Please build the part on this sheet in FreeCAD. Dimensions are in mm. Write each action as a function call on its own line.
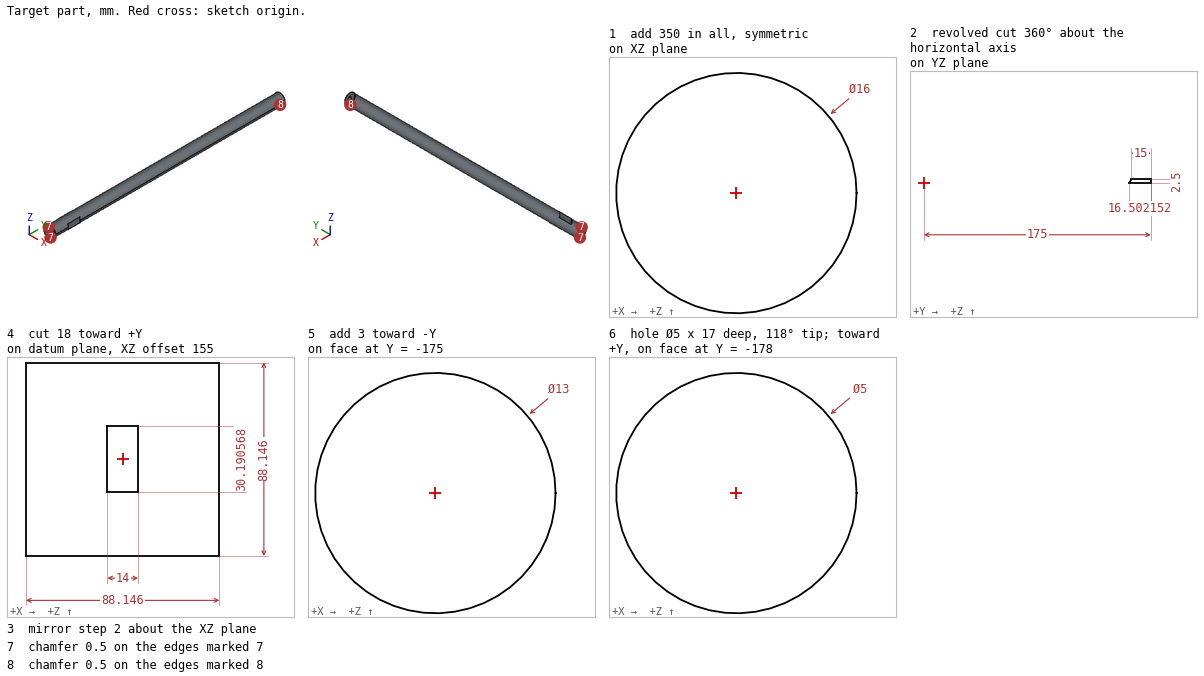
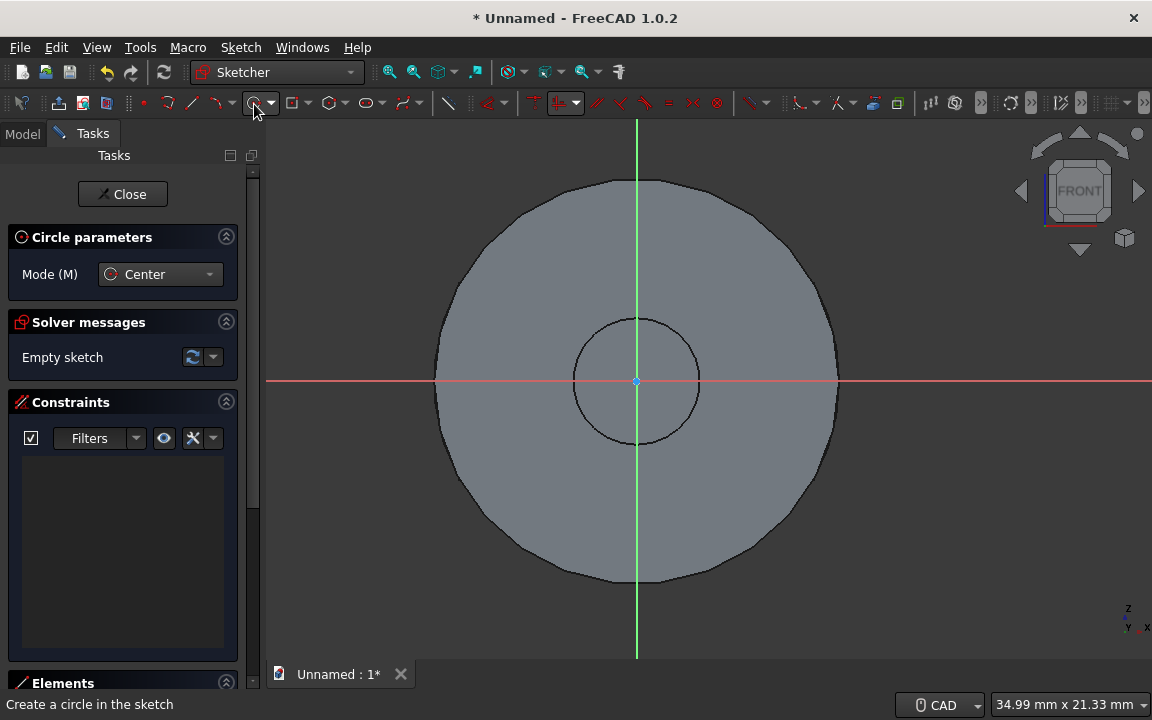
click(637, 381)
move(753, 265)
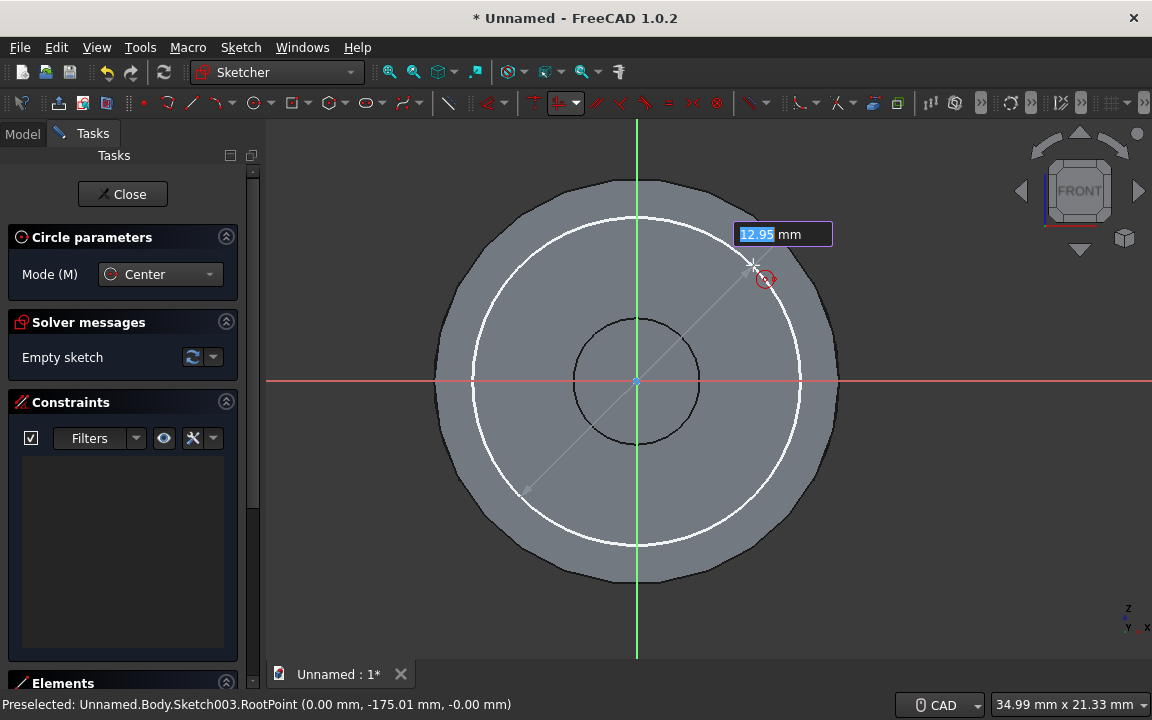
text(13)
key(Return)
key(Escape)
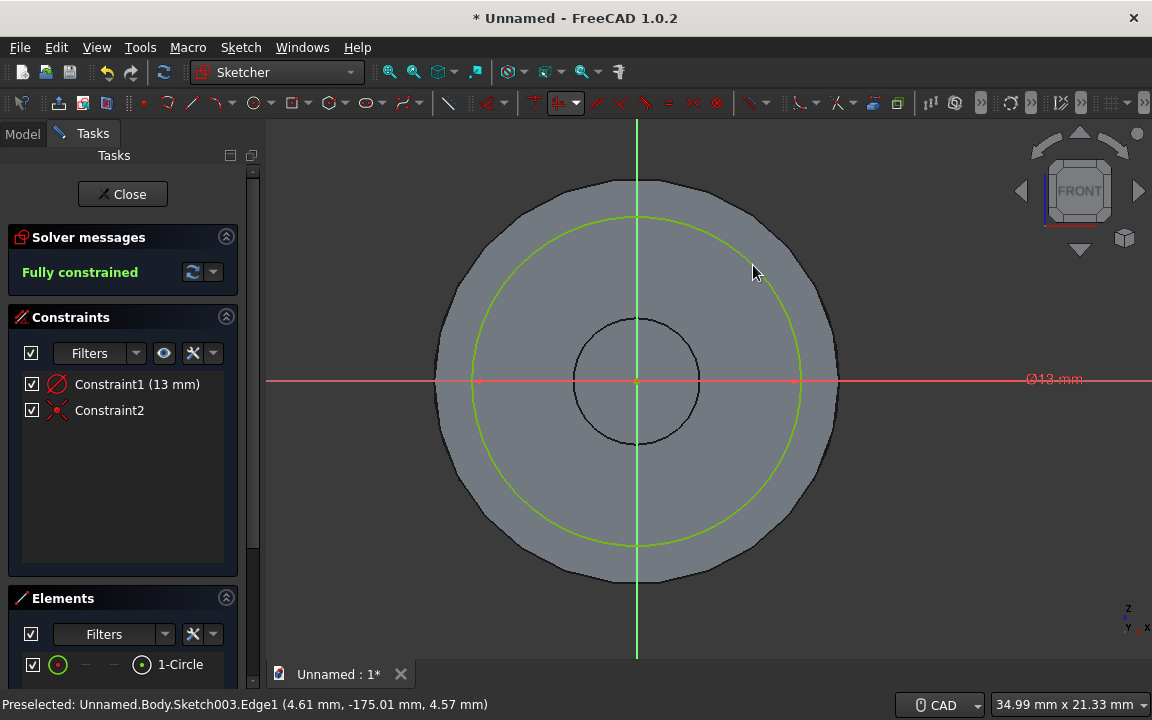
click(123, 194)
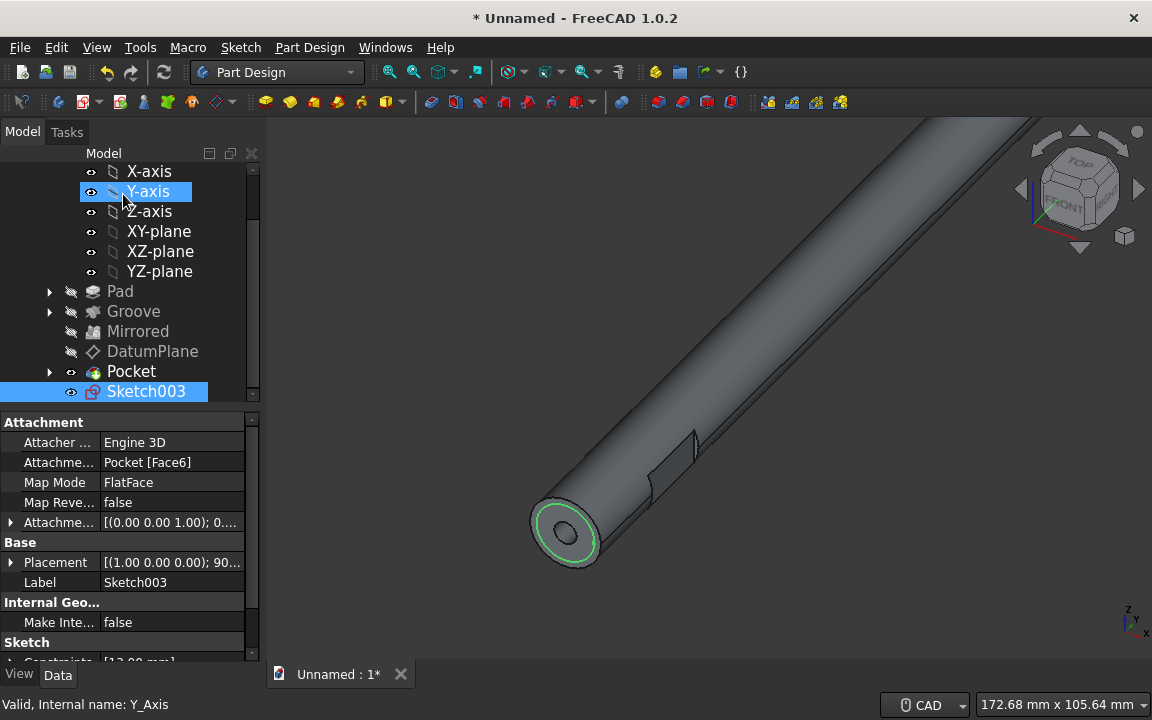
click(266, 102)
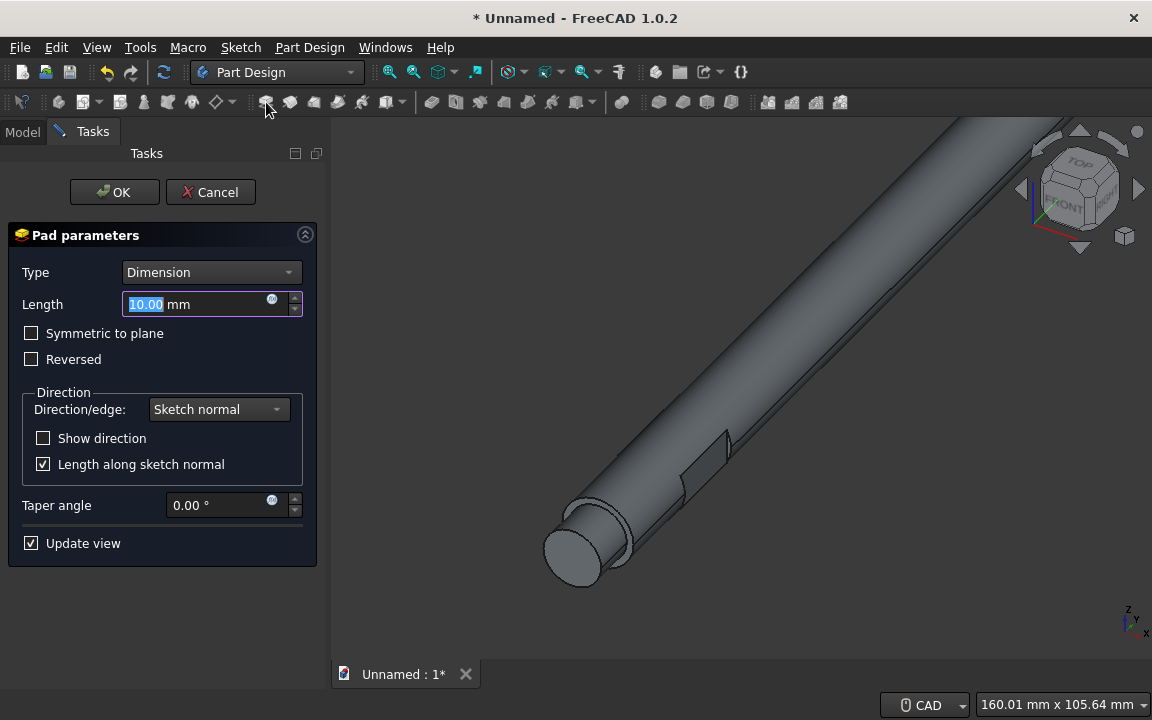
text(3)
key(Tab)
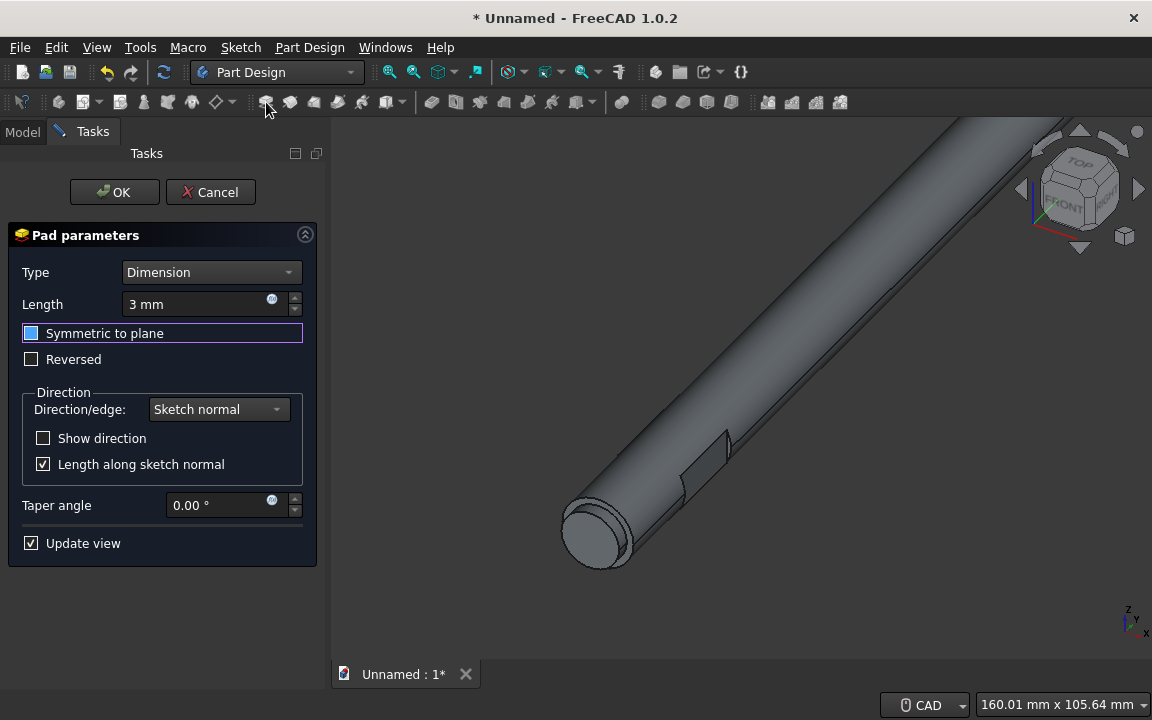
click(115, 192)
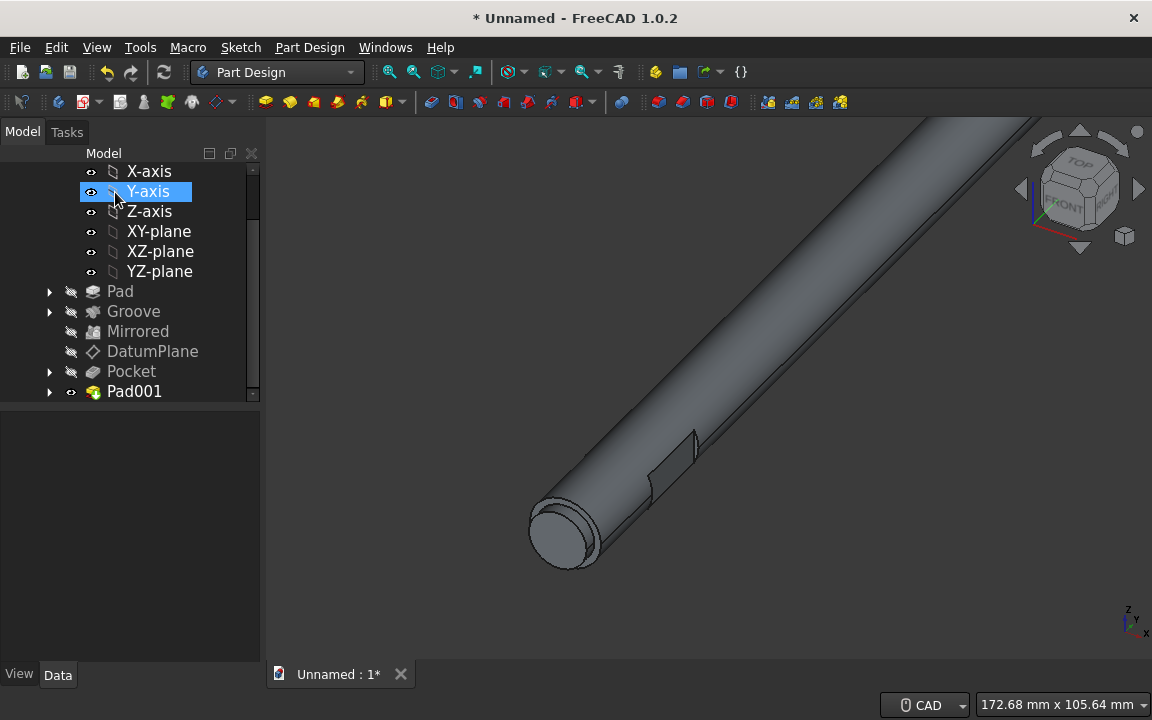
click(390, 72)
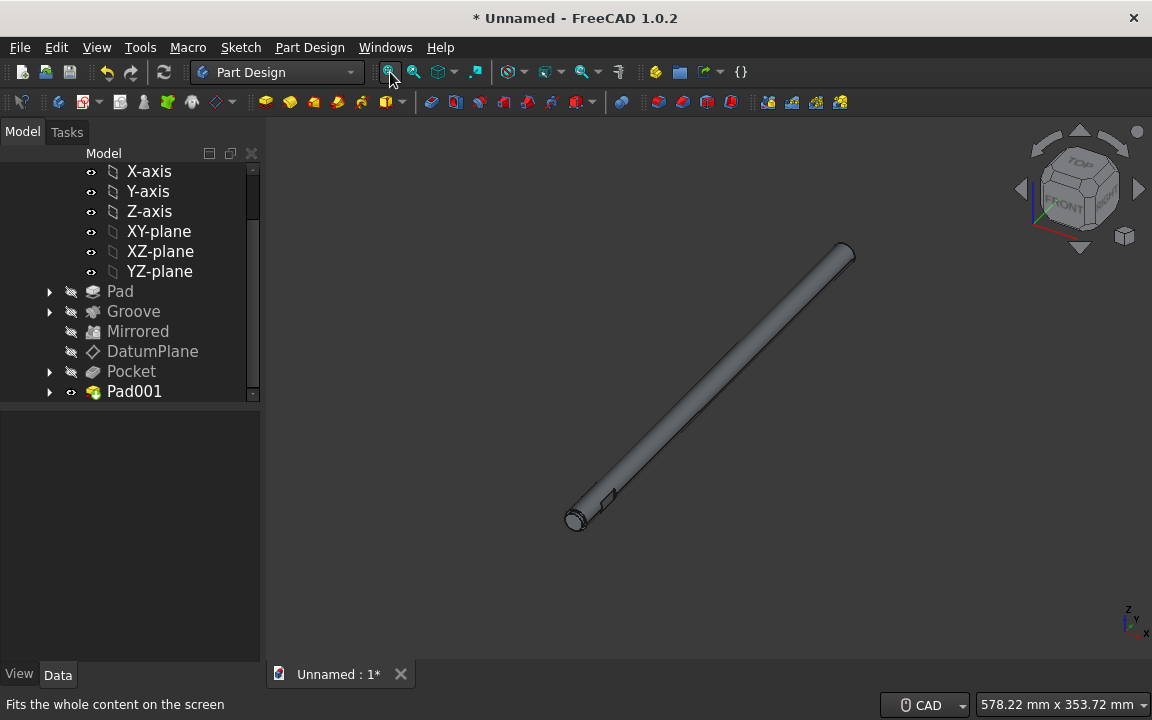
key(0)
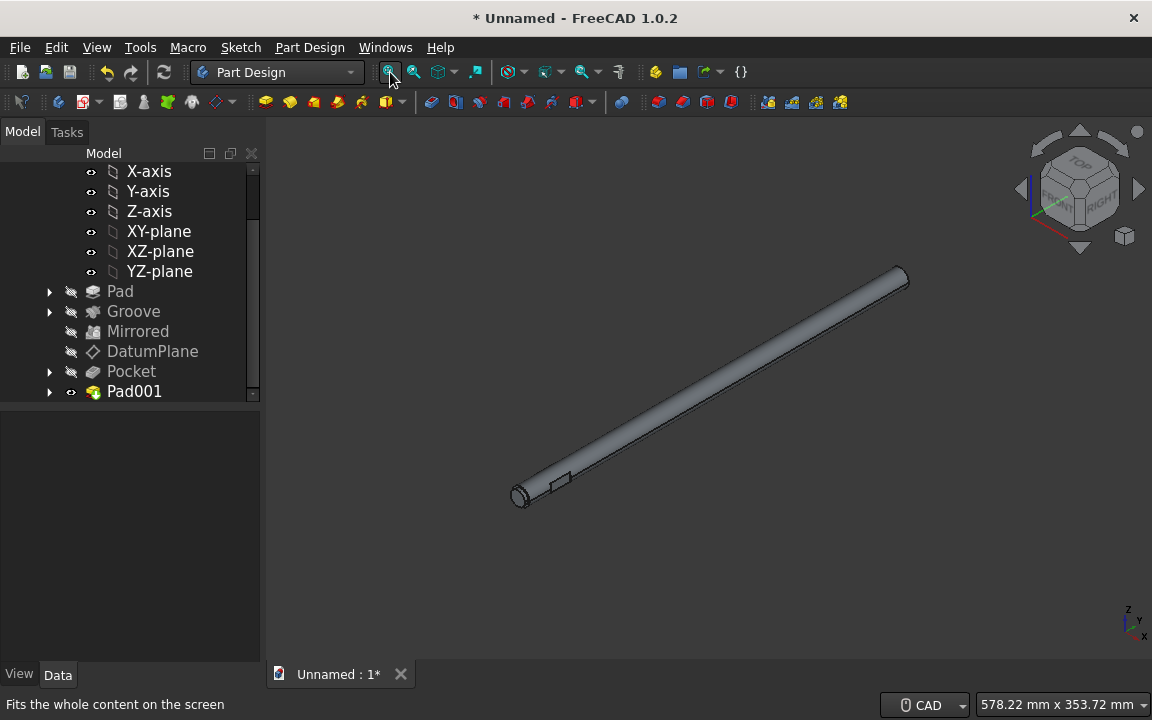
key(1)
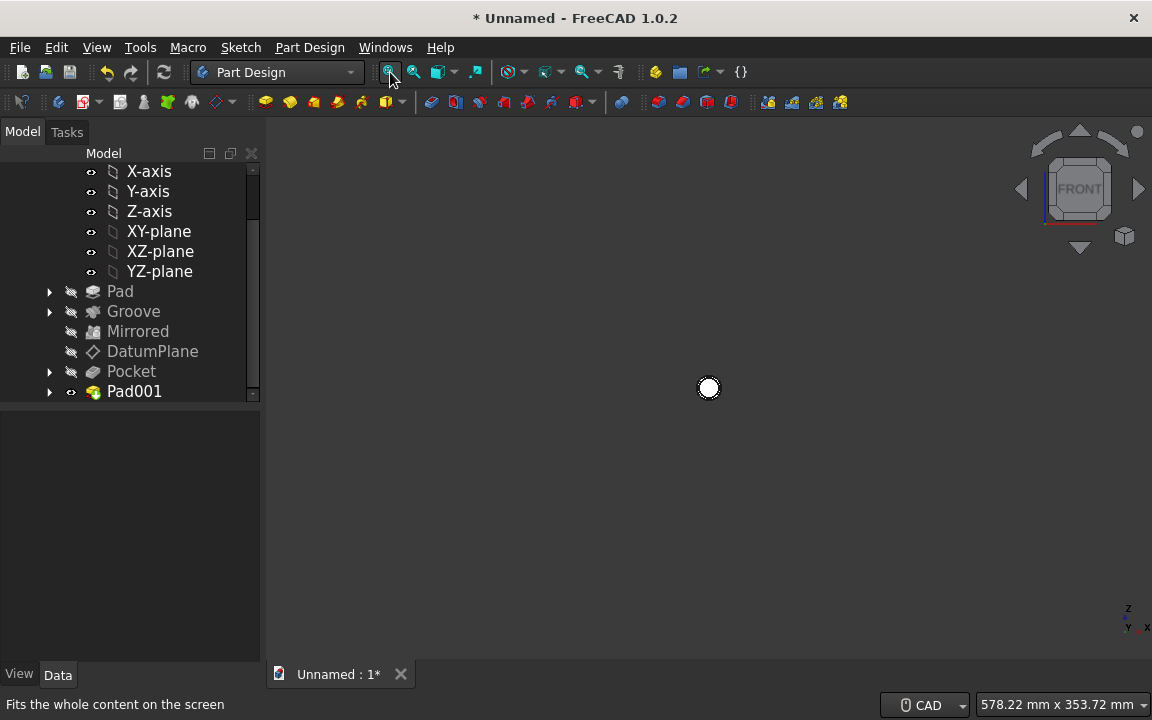
click(390, 72)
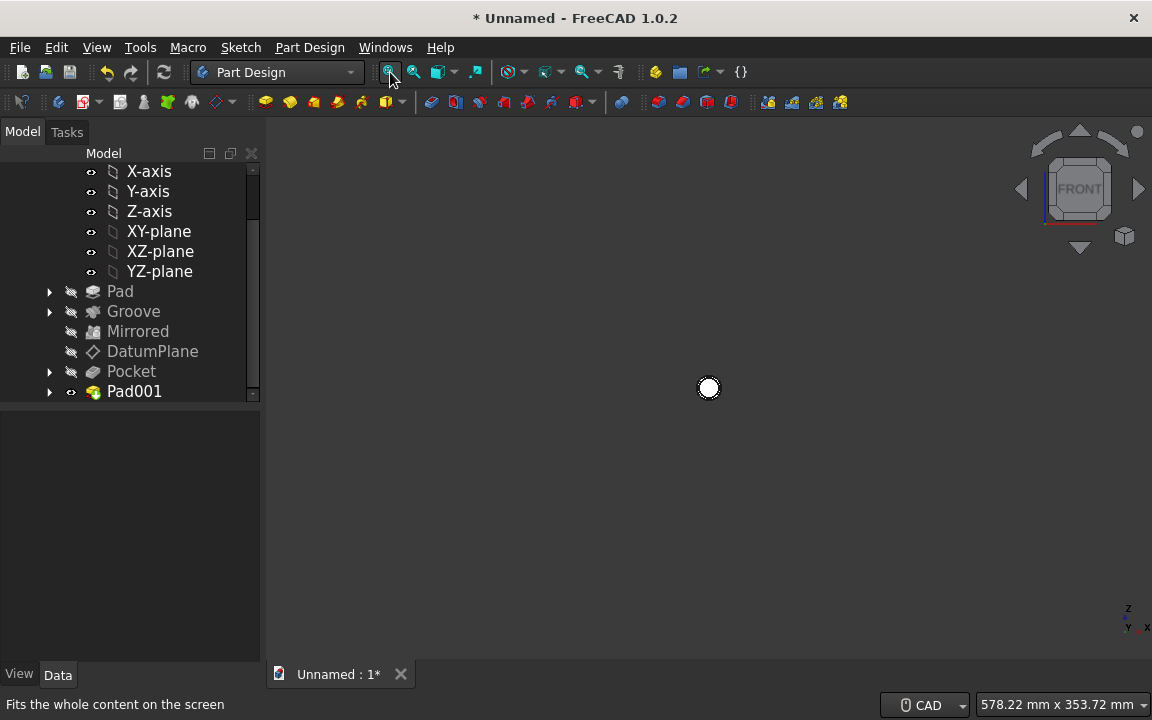
click(709, 387)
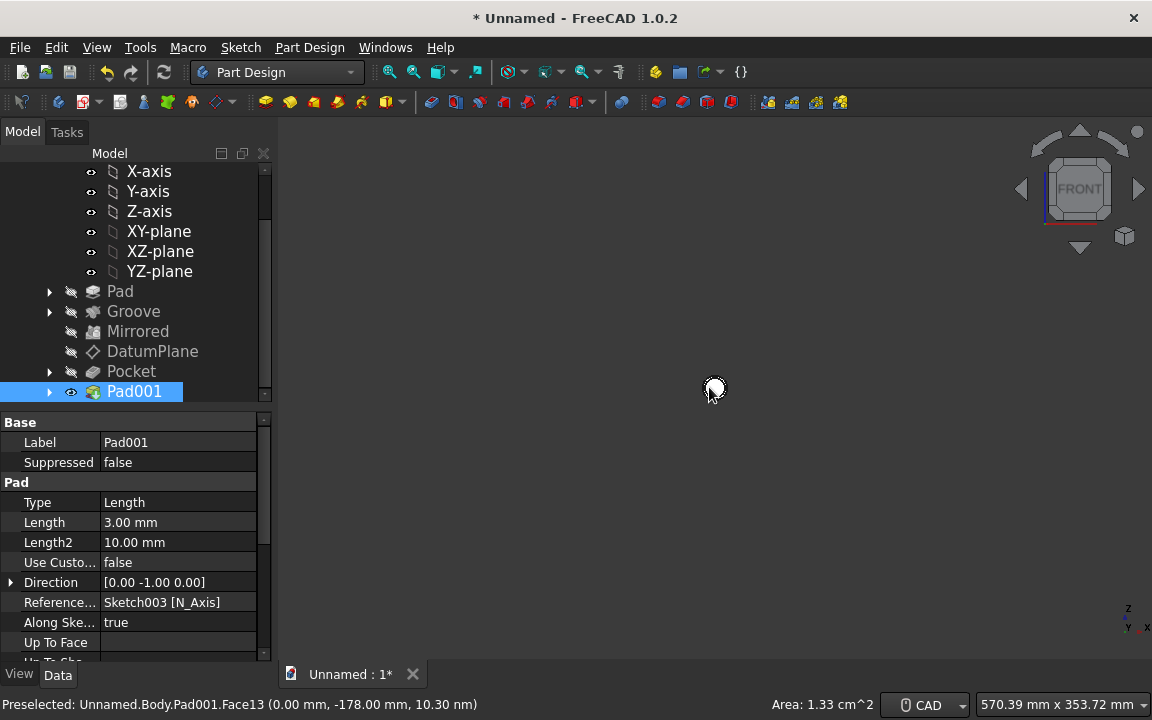
click(84, 102)